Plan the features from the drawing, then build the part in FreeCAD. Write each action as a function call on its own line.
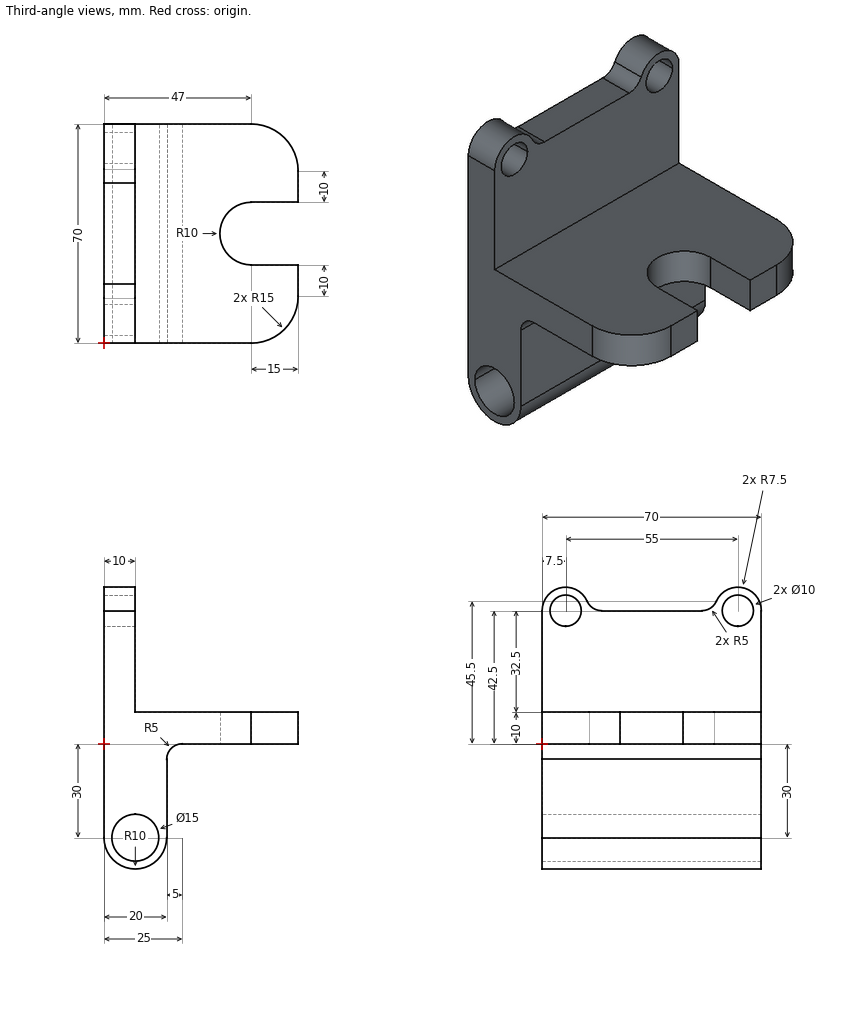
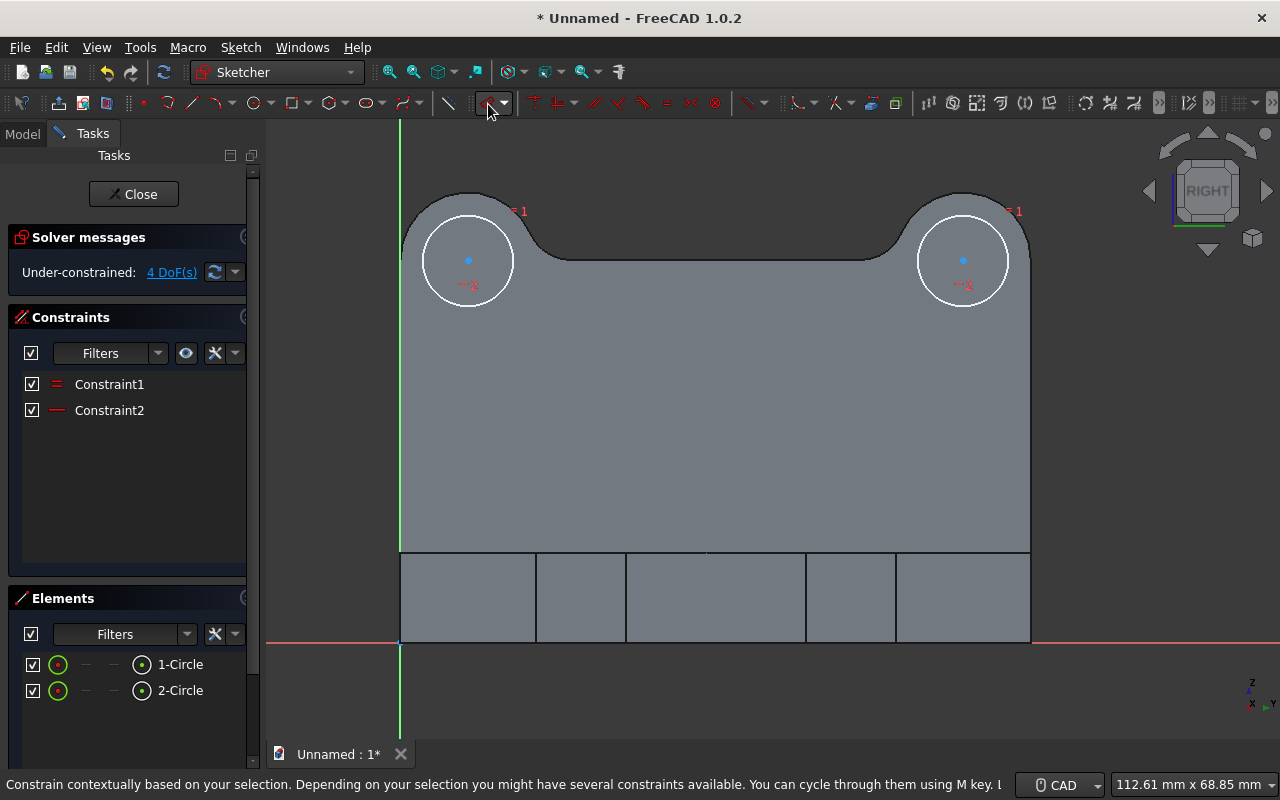
click(995, 229)
click(1018, 206)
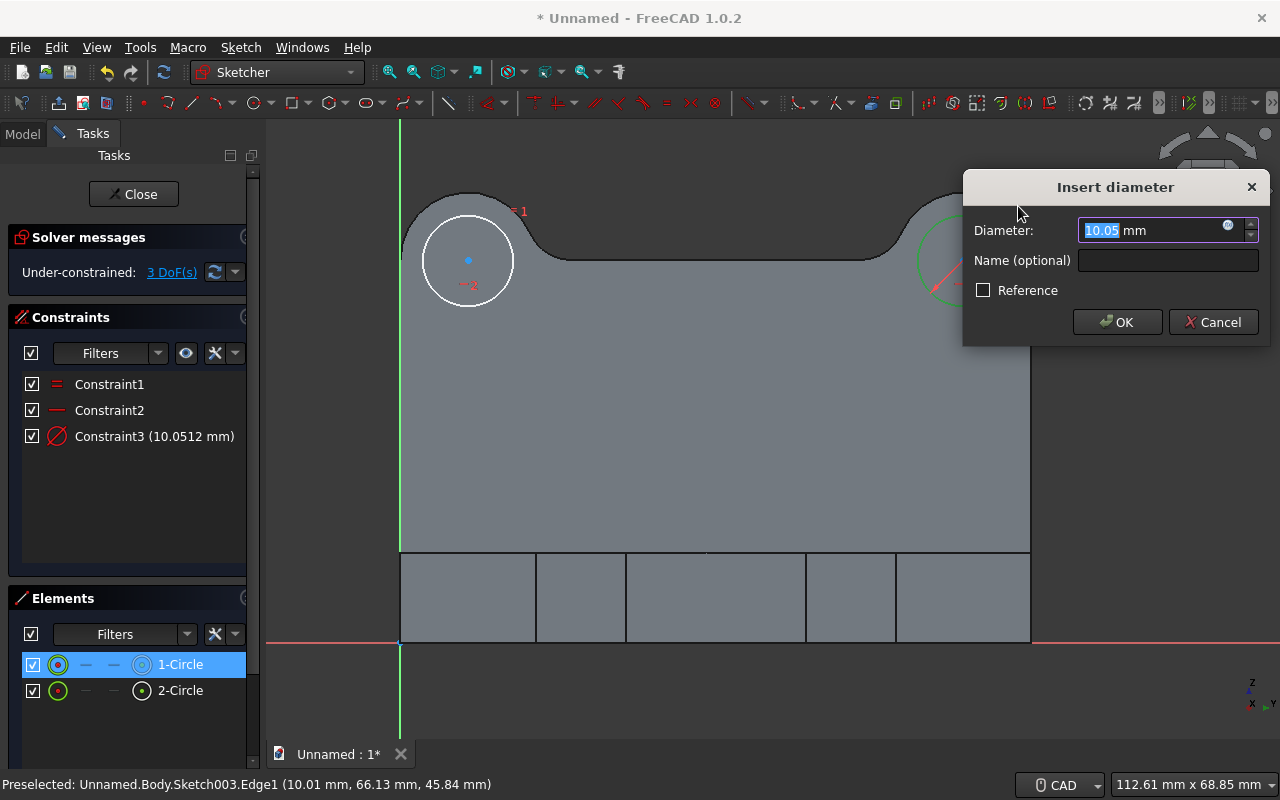
text(10)
key(Return)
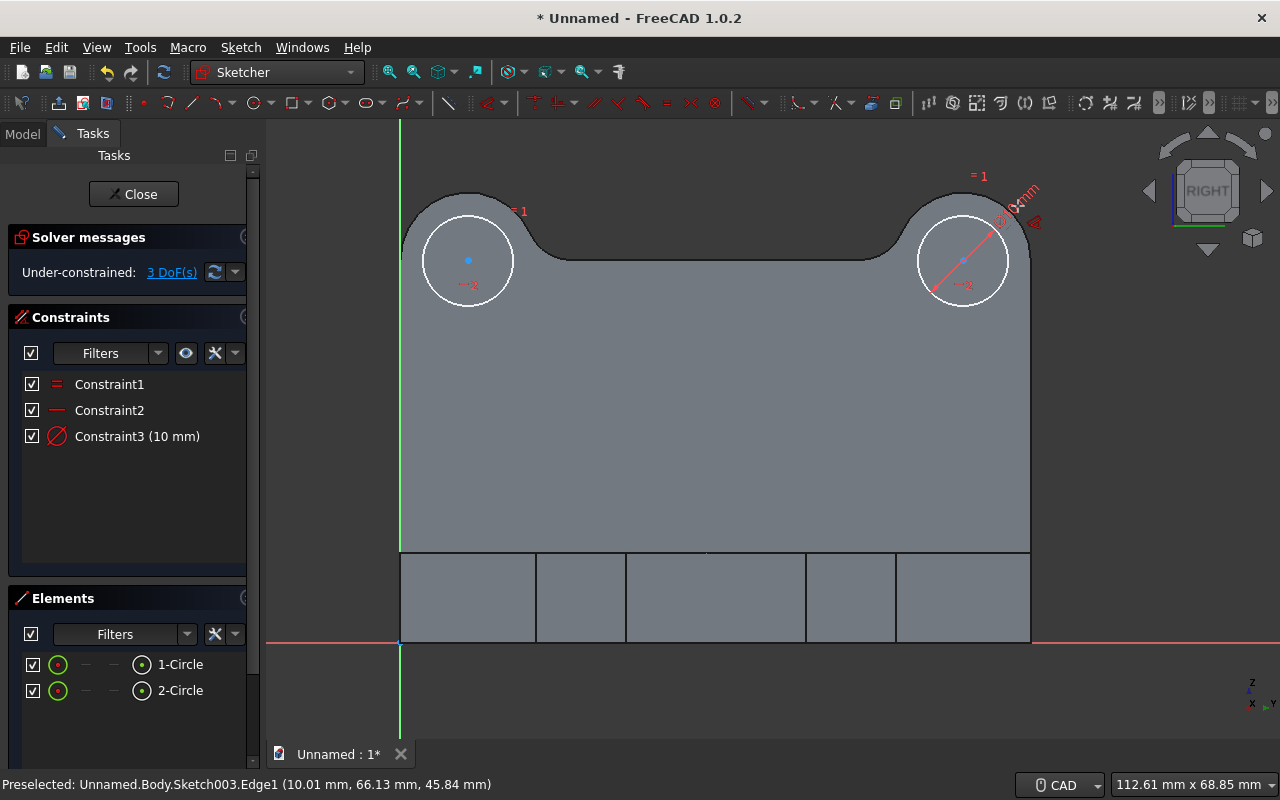
click(468, 261)
click(434, 677)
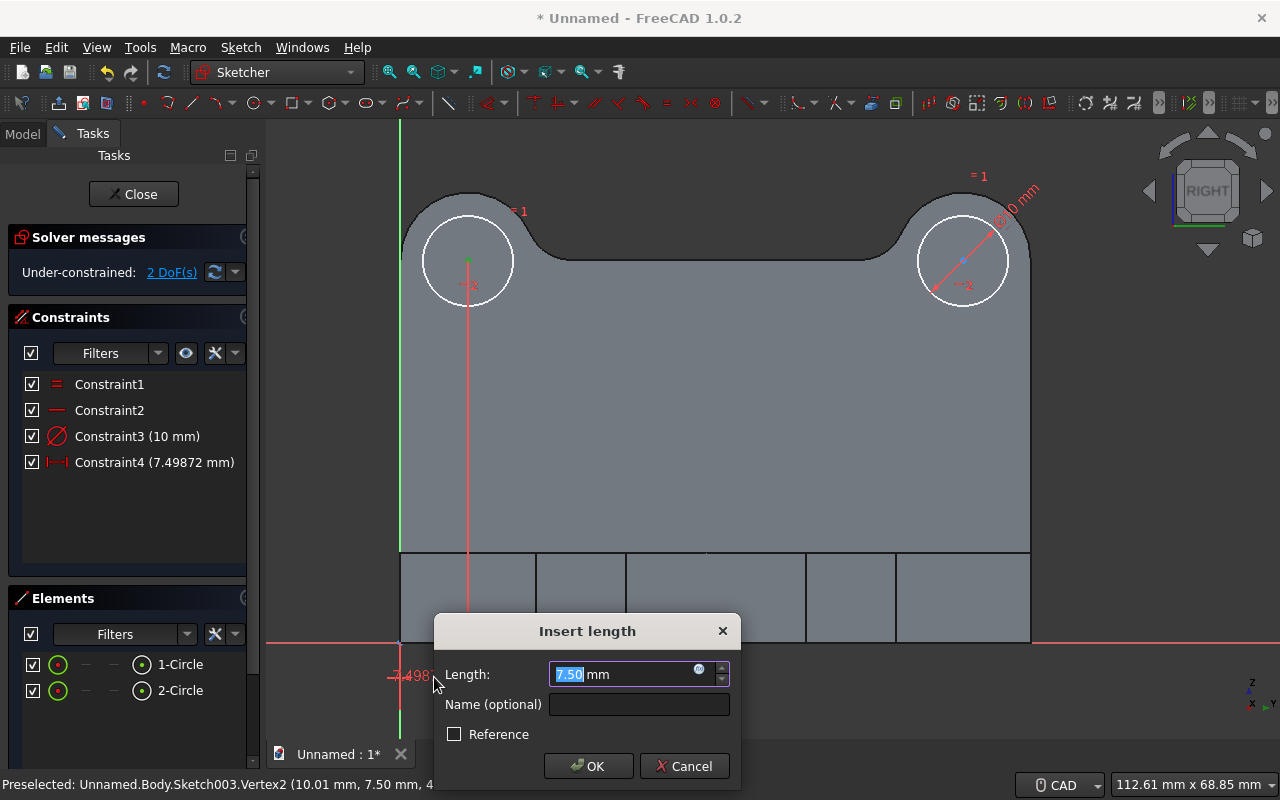
text(7.5)
key(Return)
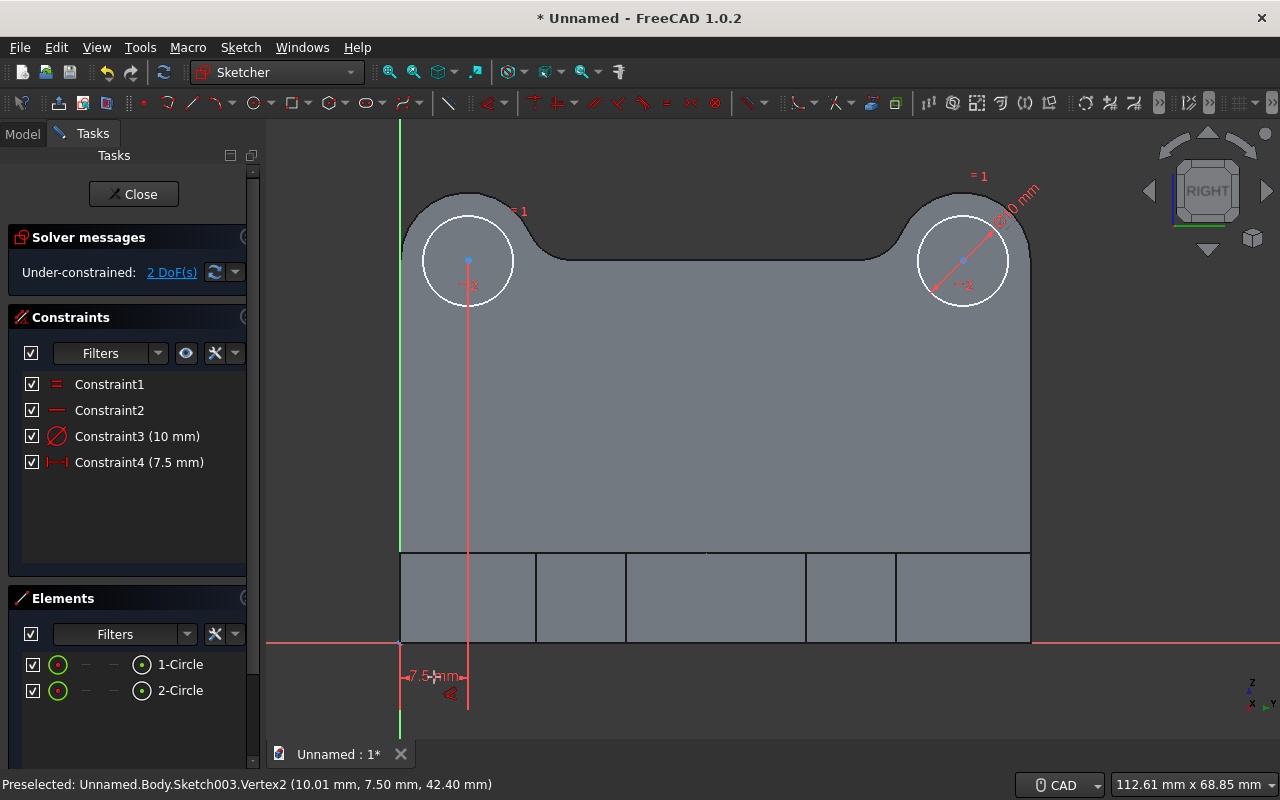
click(963, 261)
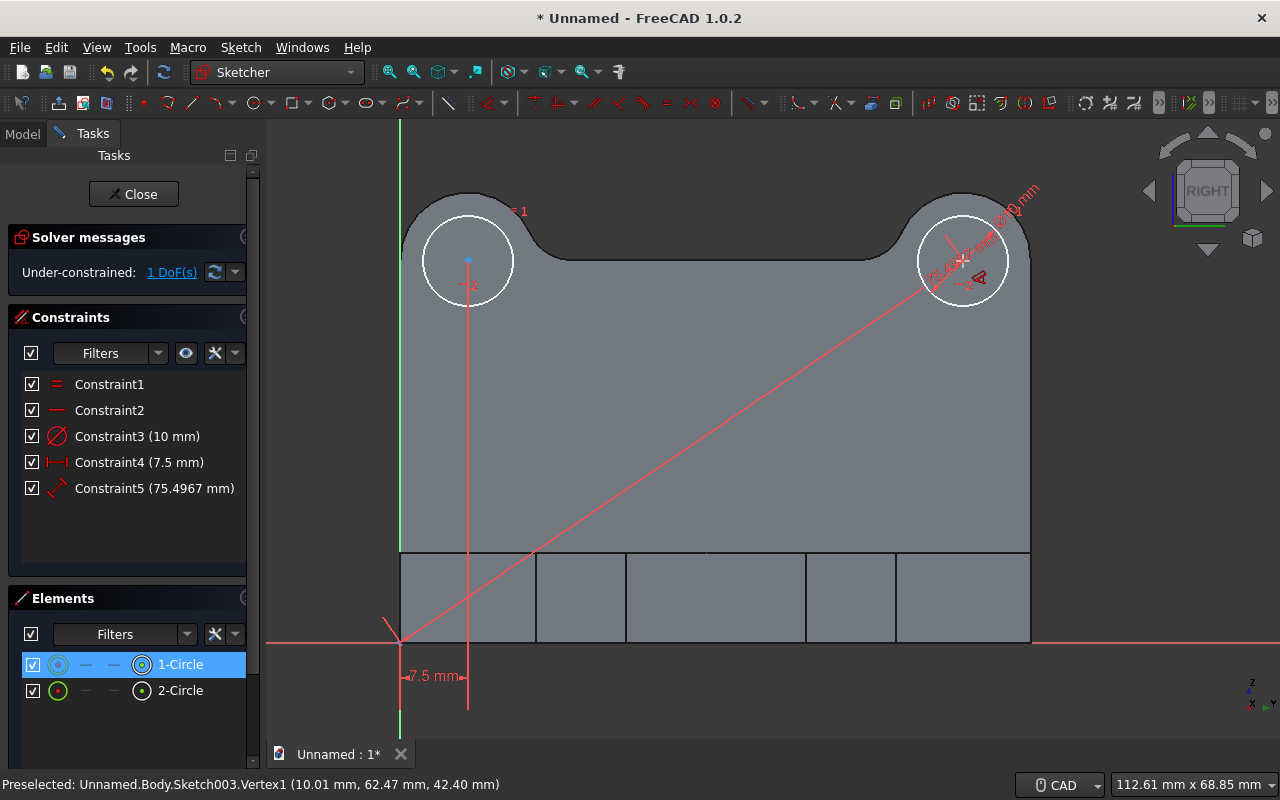
click(468, 261)
click(716, 227)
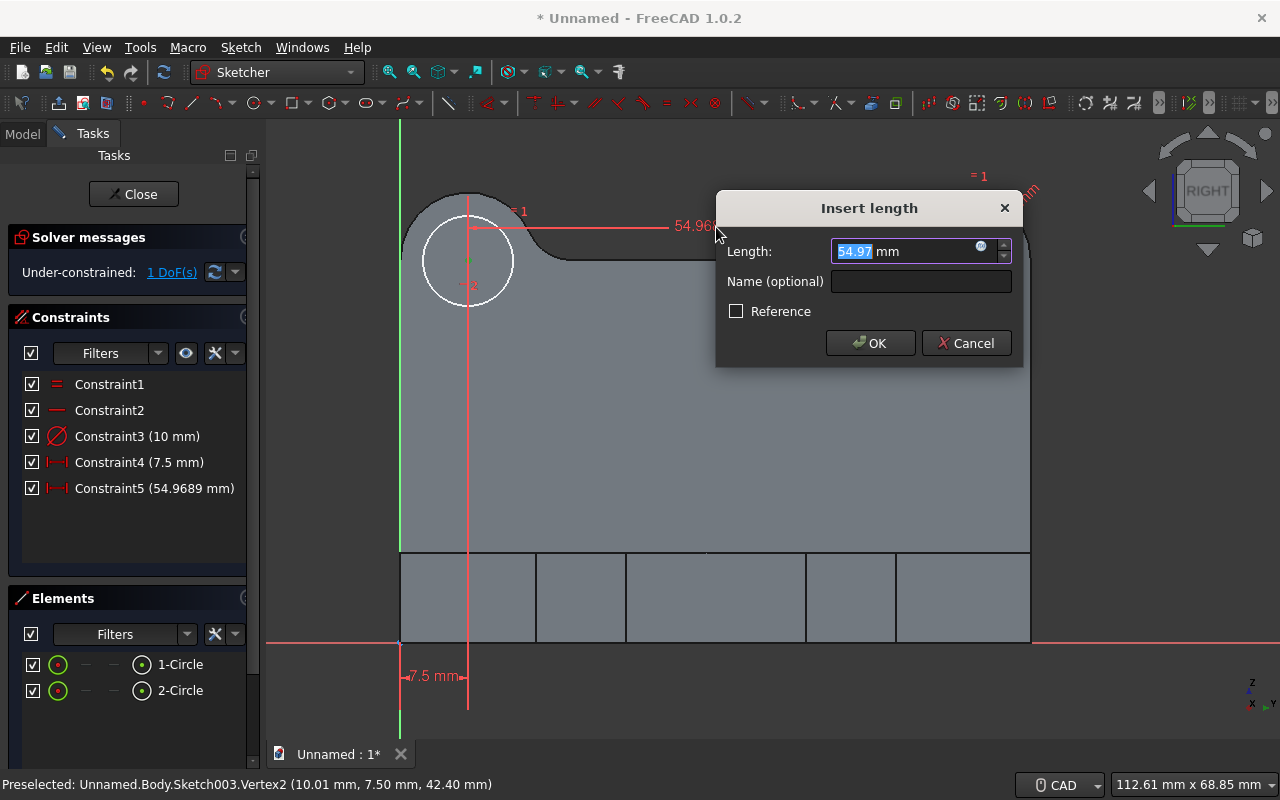
text(55)
key(Return)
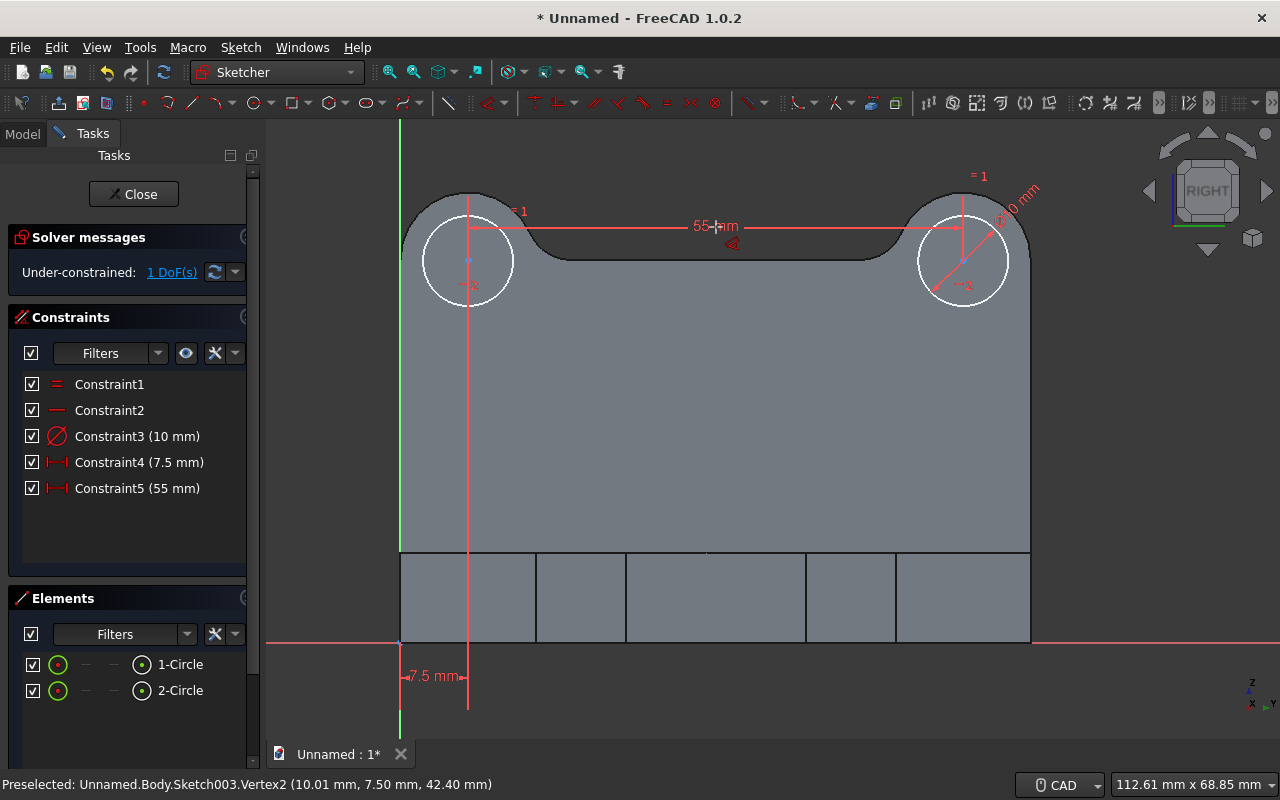
click(963, 261)
click(366, 452)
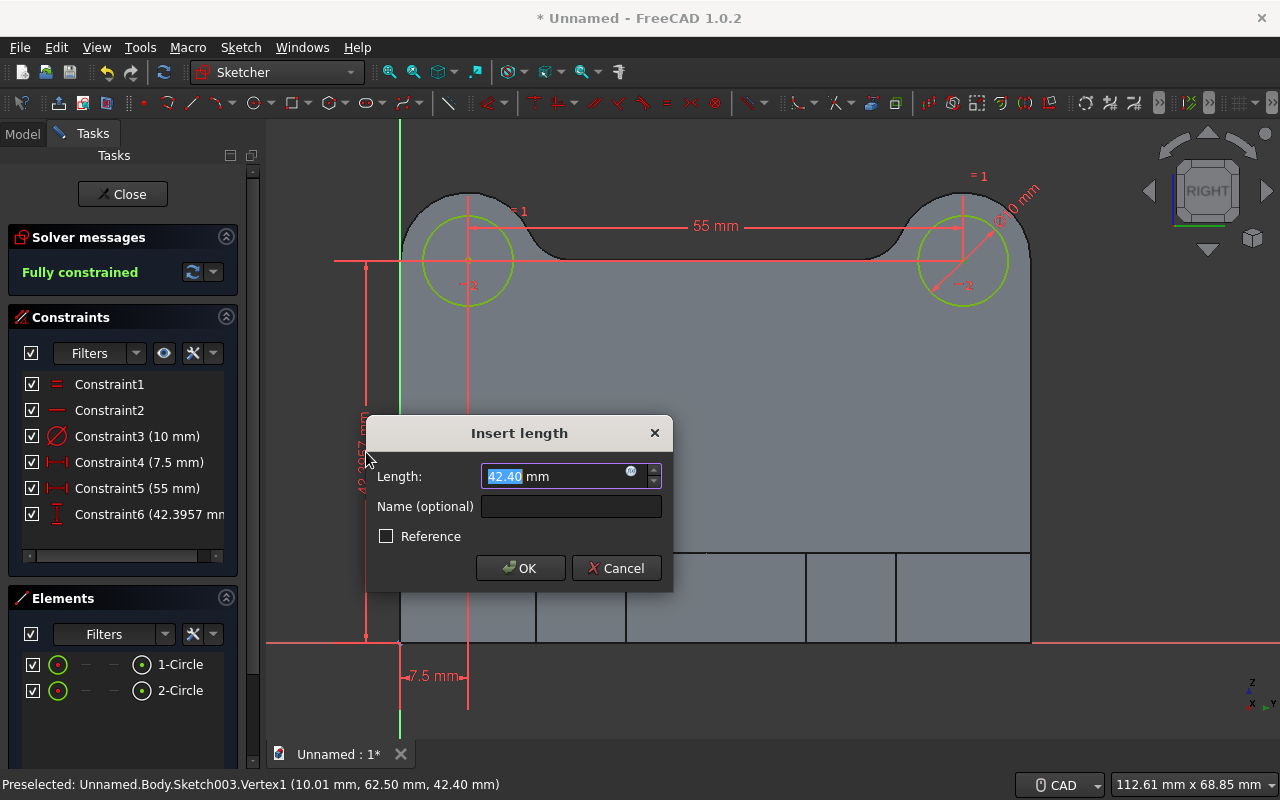
text(42.5)
key(Return)
key(Escape)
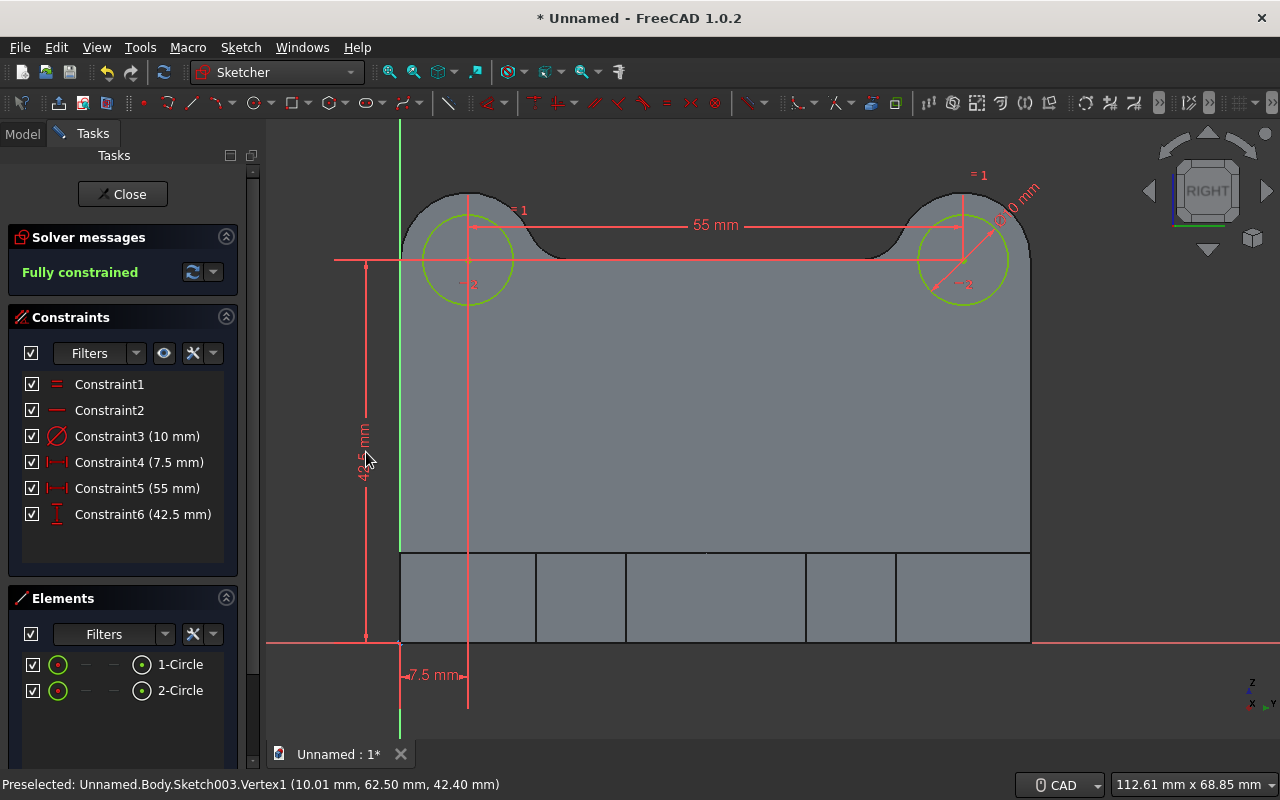
click(123, 194)